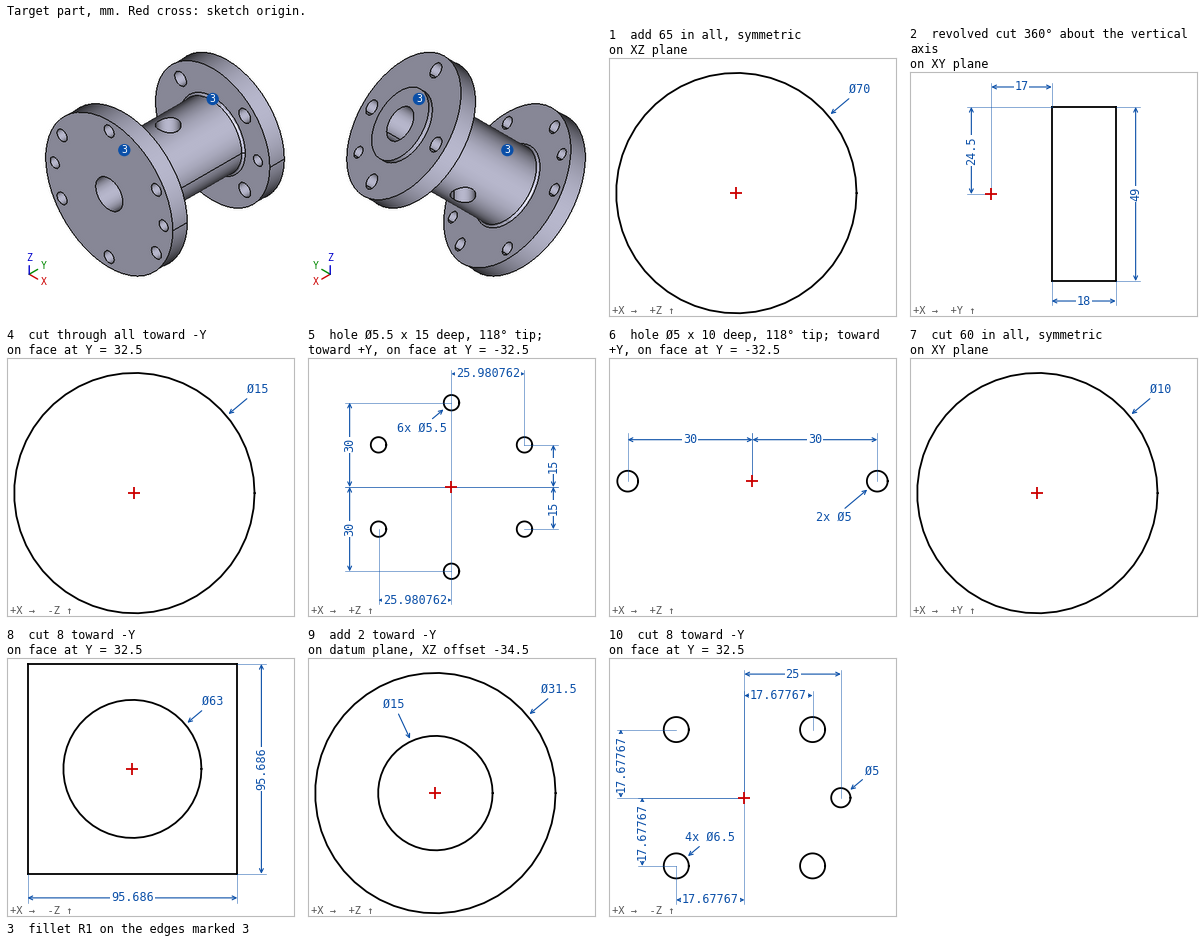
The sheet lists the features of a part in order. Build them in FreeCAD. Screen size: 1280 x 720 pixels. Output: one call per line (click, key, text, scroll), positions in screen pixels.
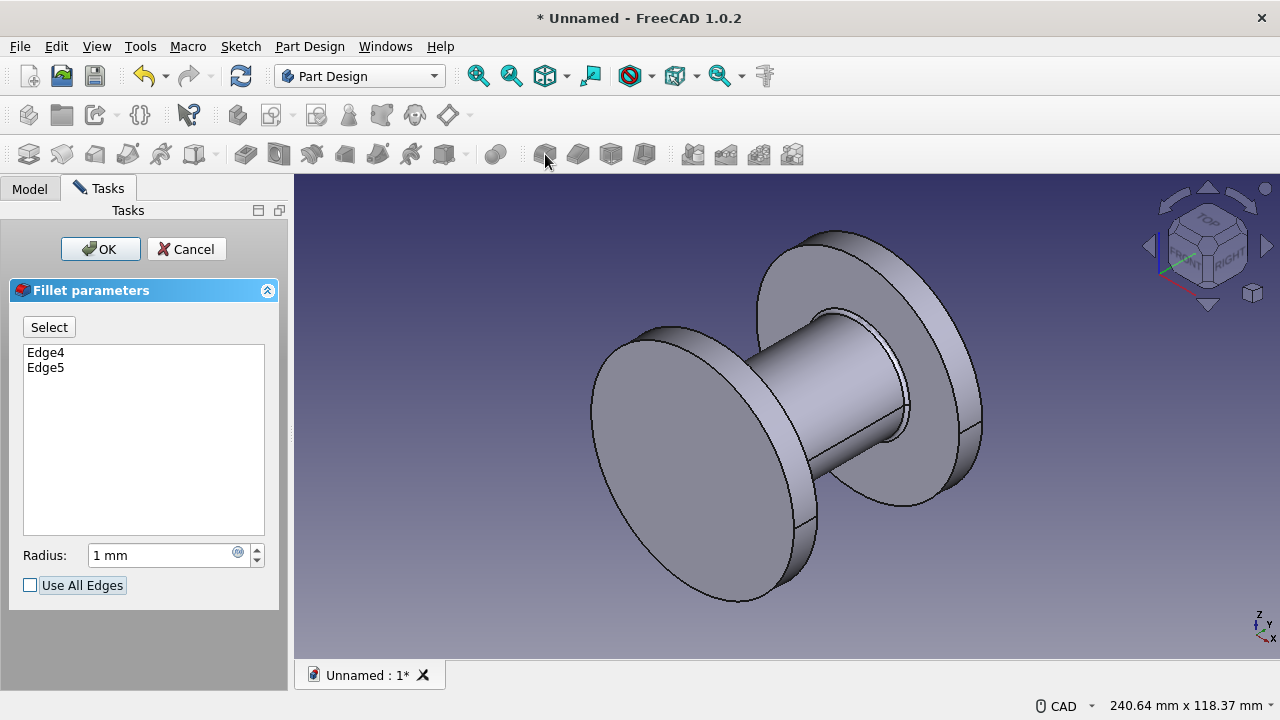
click(101, 249)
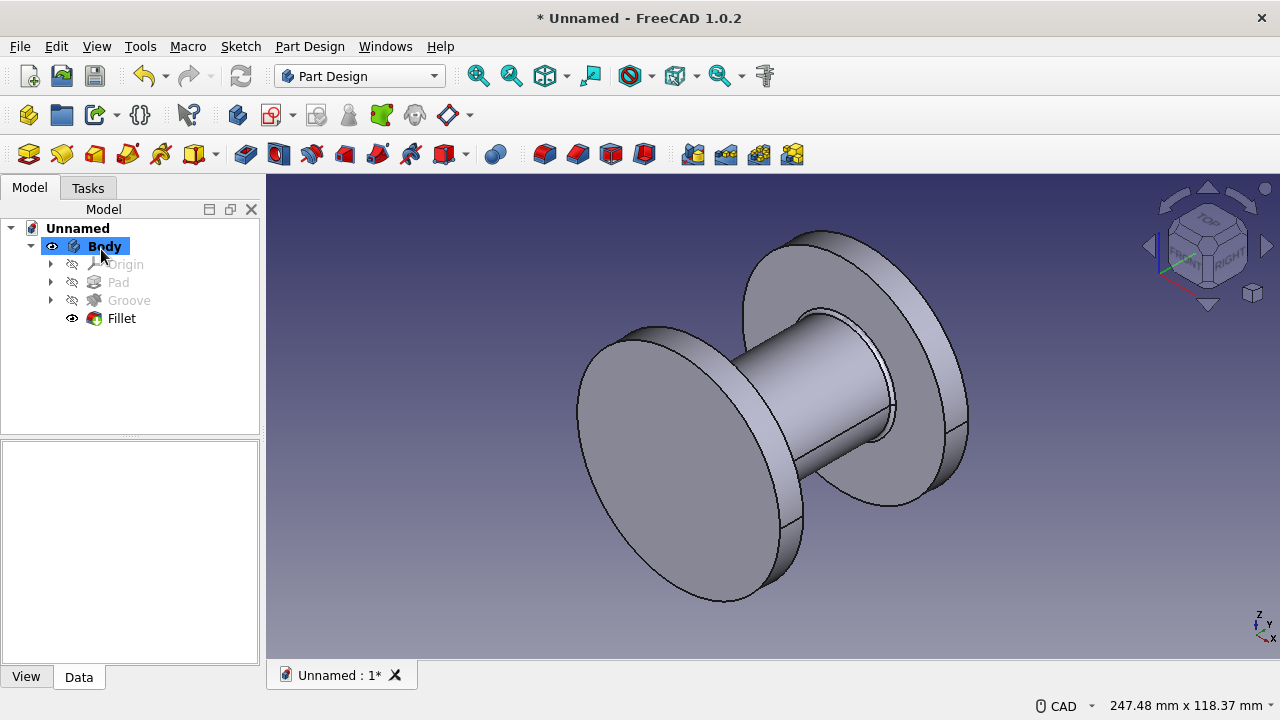
key(4)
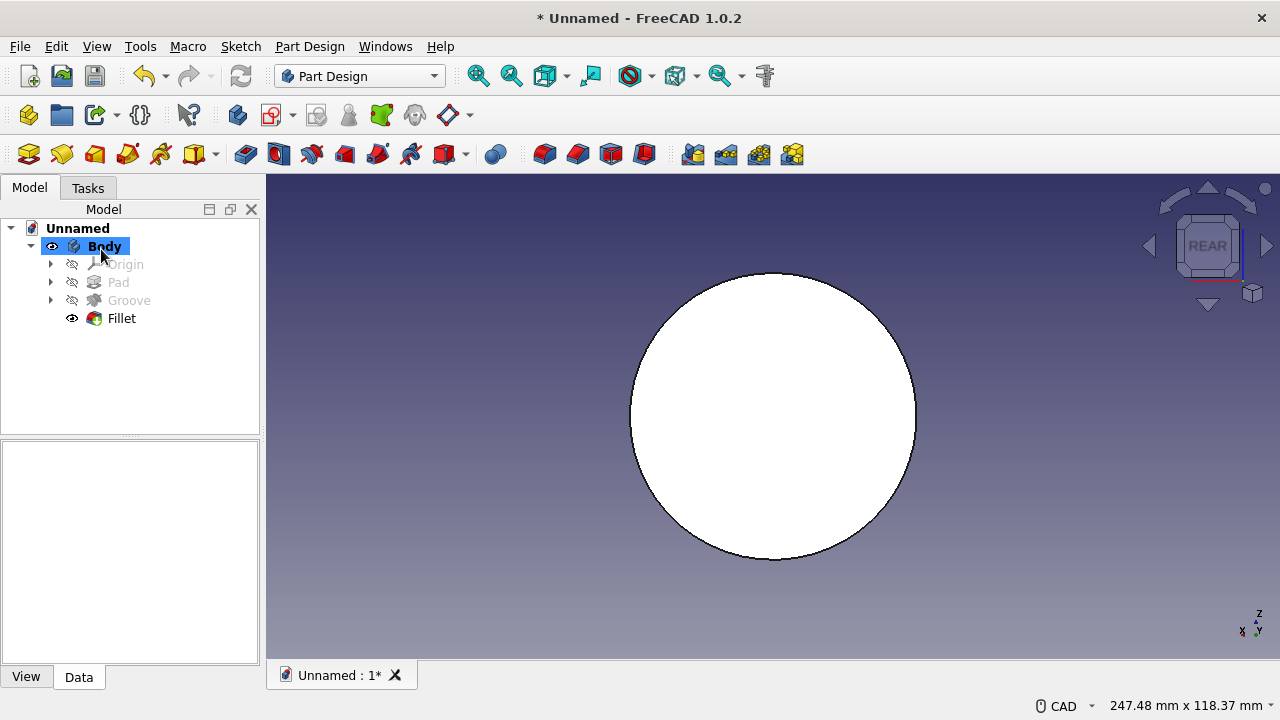
click(773, 415)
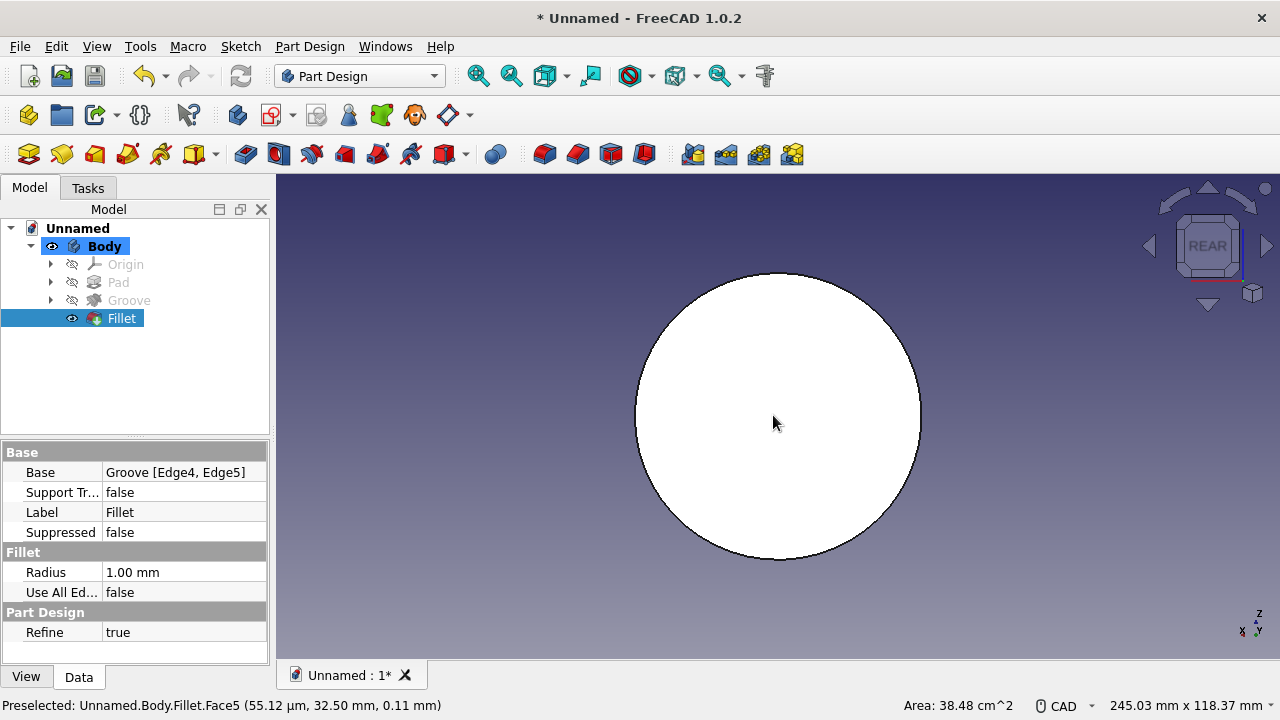
click(270, 116)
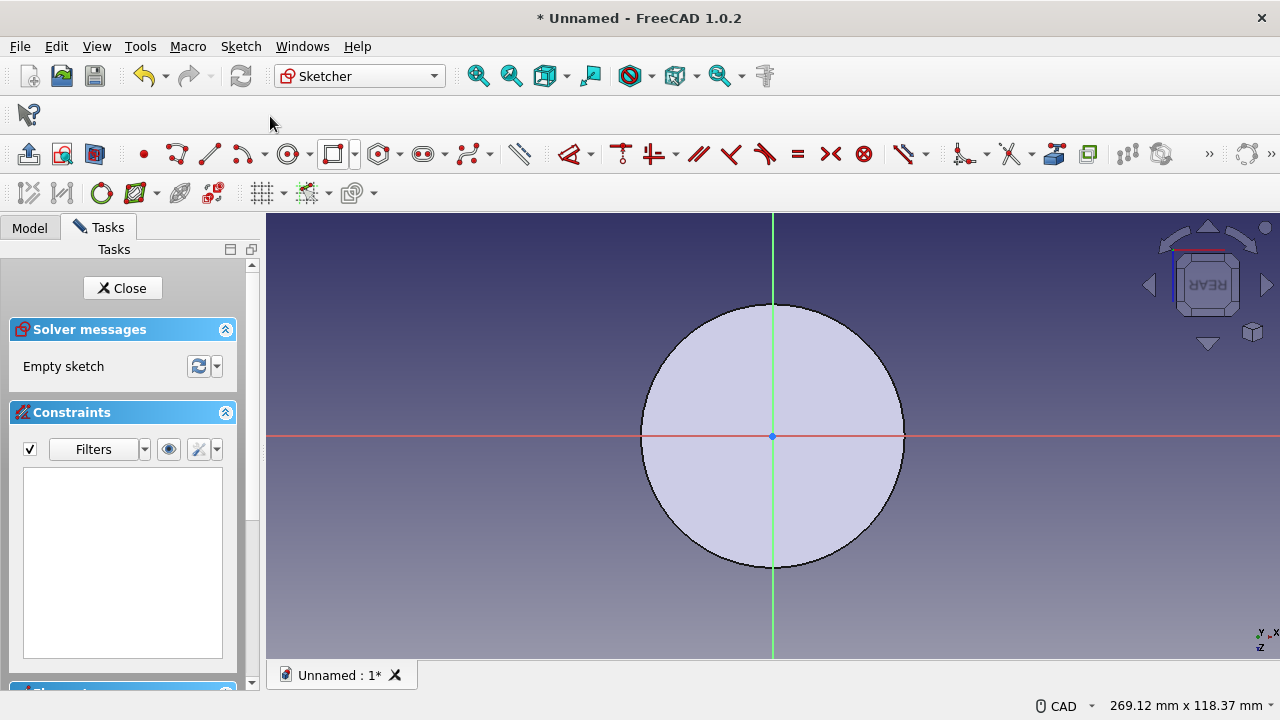
scroll(790, 436, up, 8)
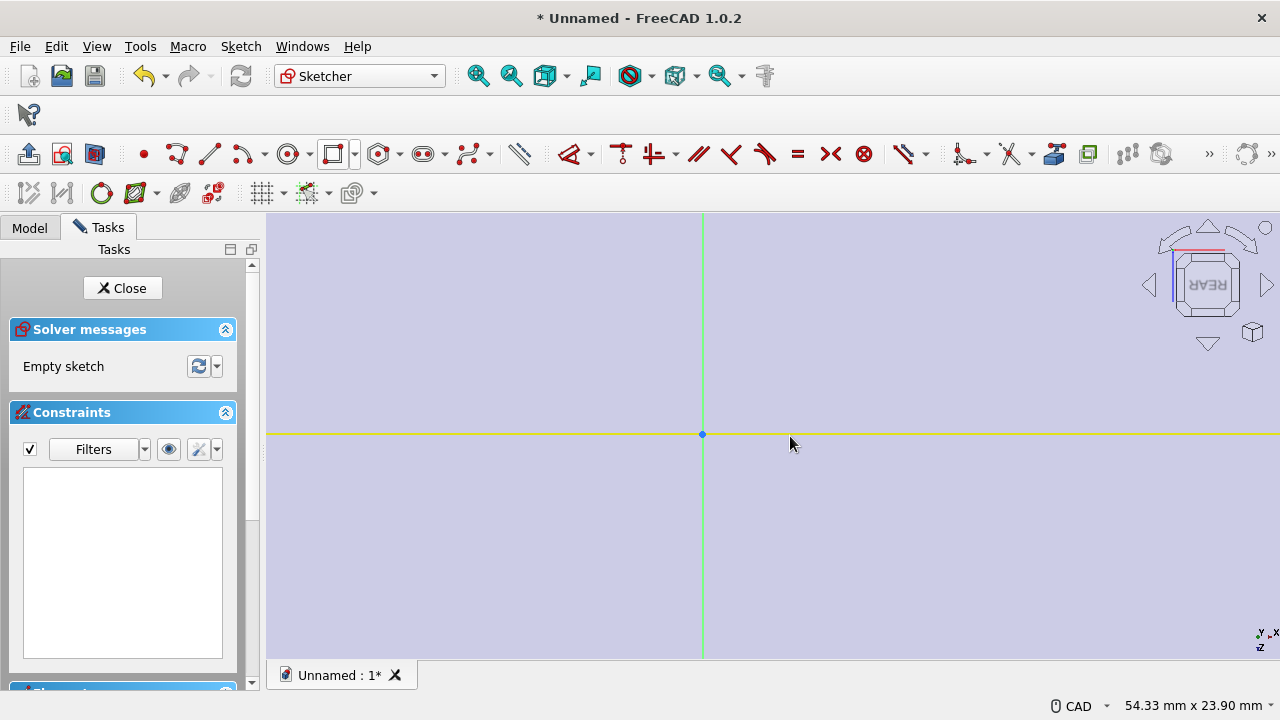
click(288, 154)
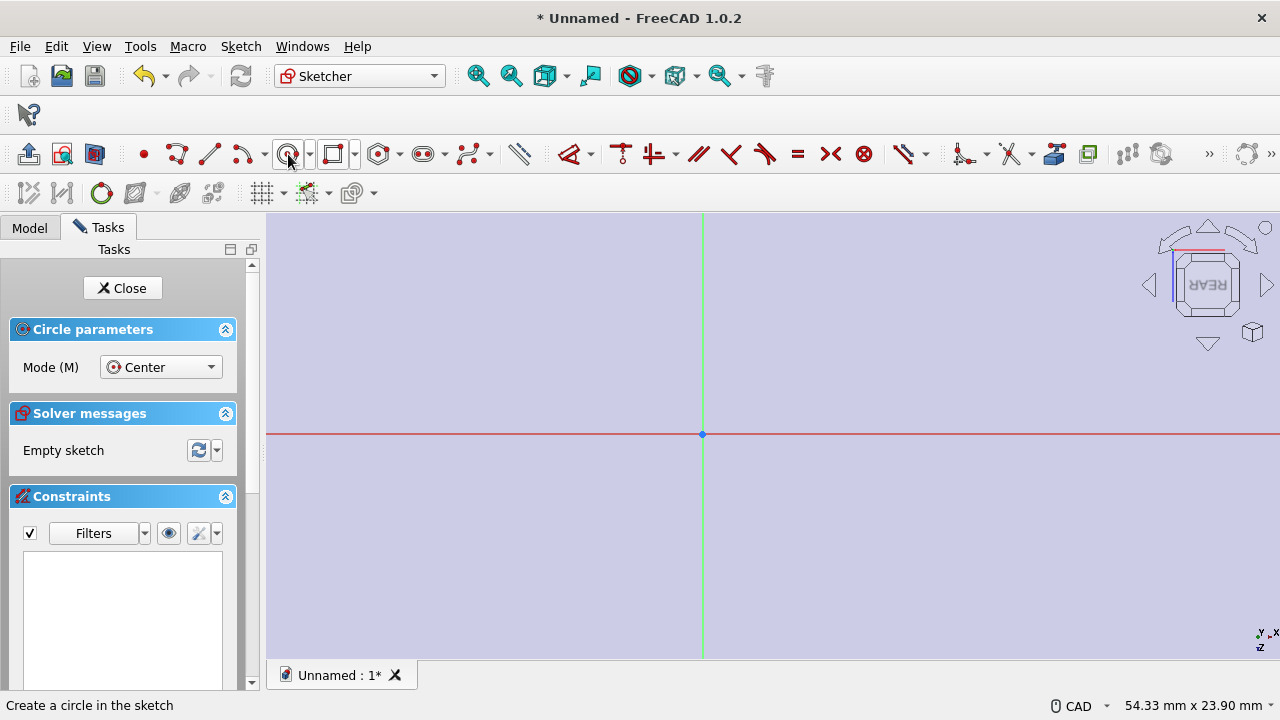
click(703, 434)
move(802, 335)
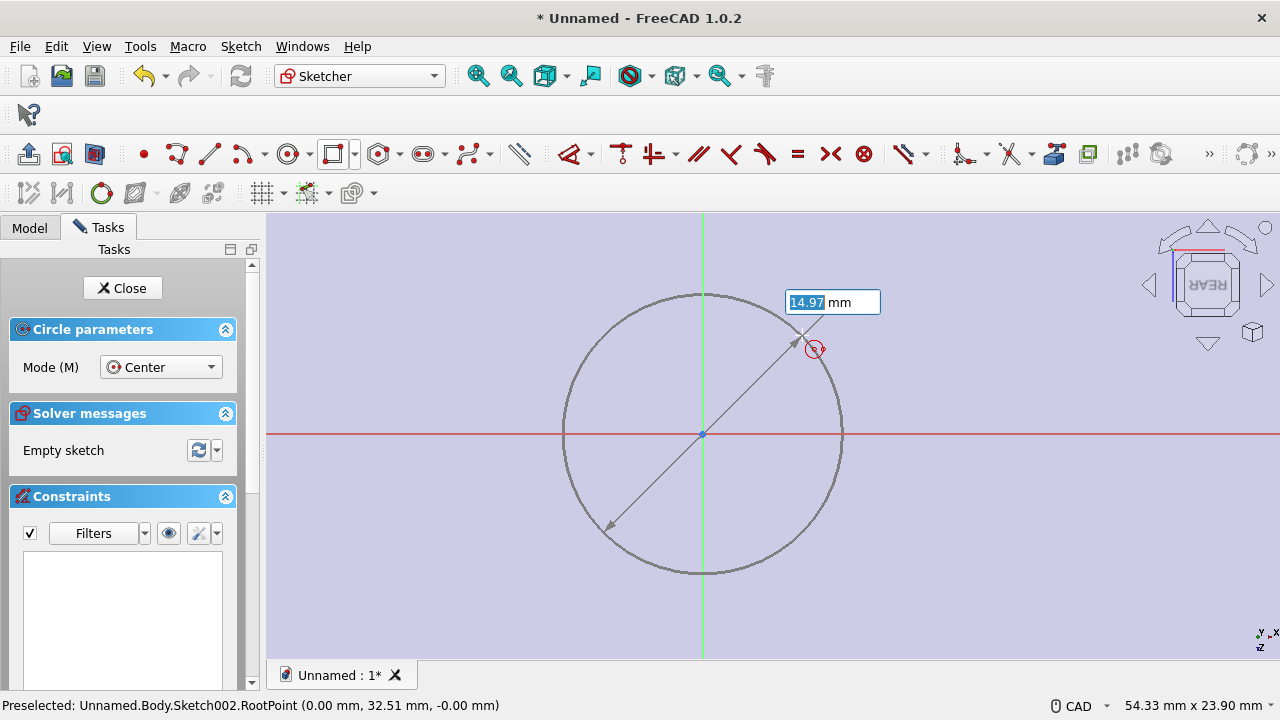
text(15)
key(Return)
key(Escape)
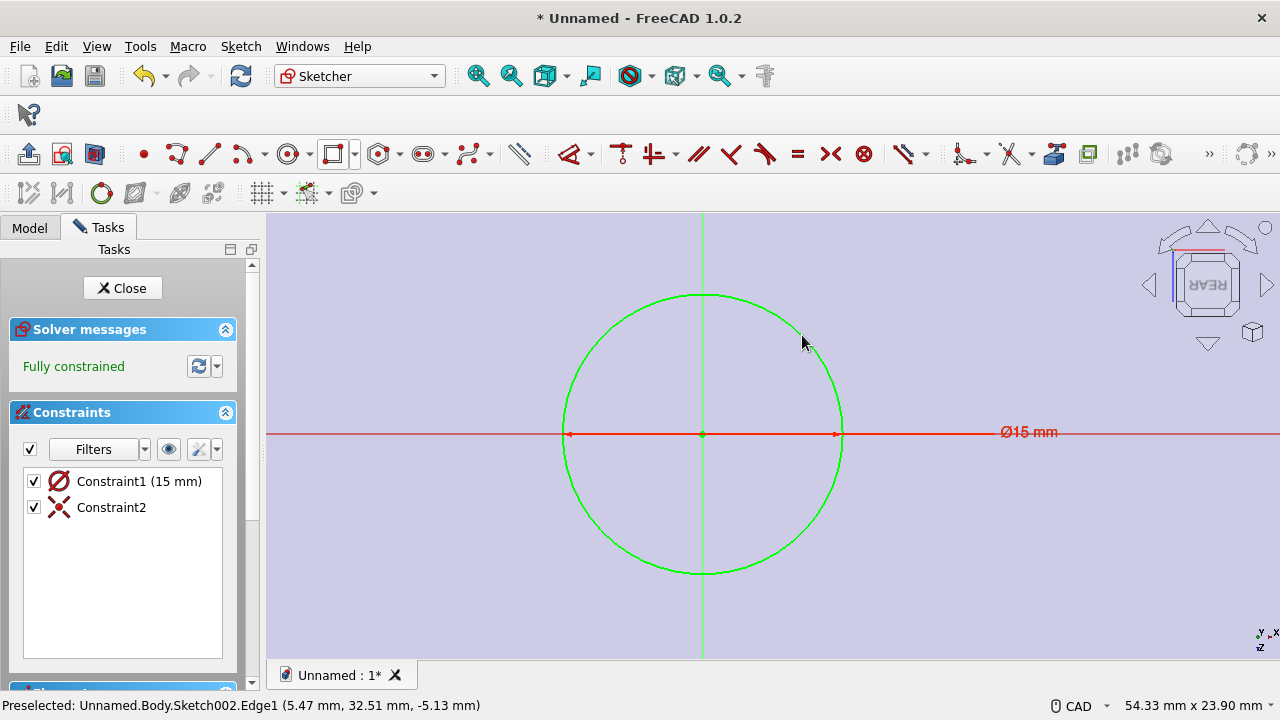
click(123, 288)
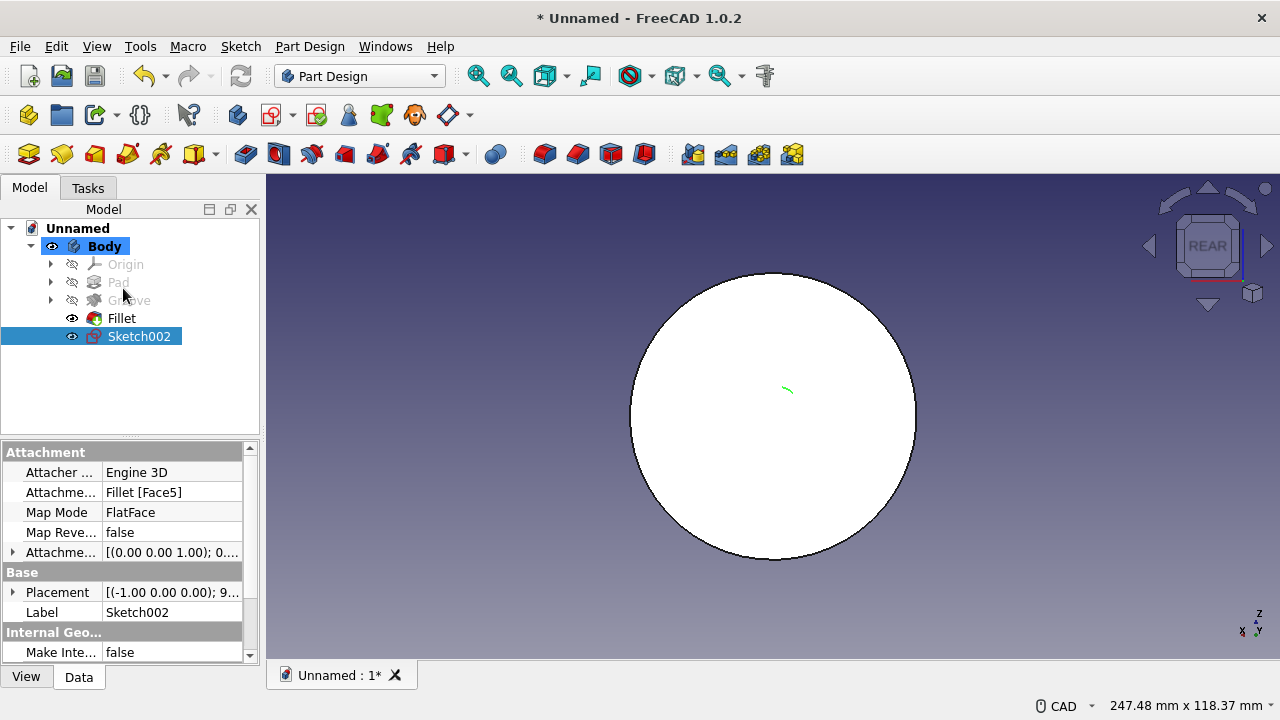
click(246, 154)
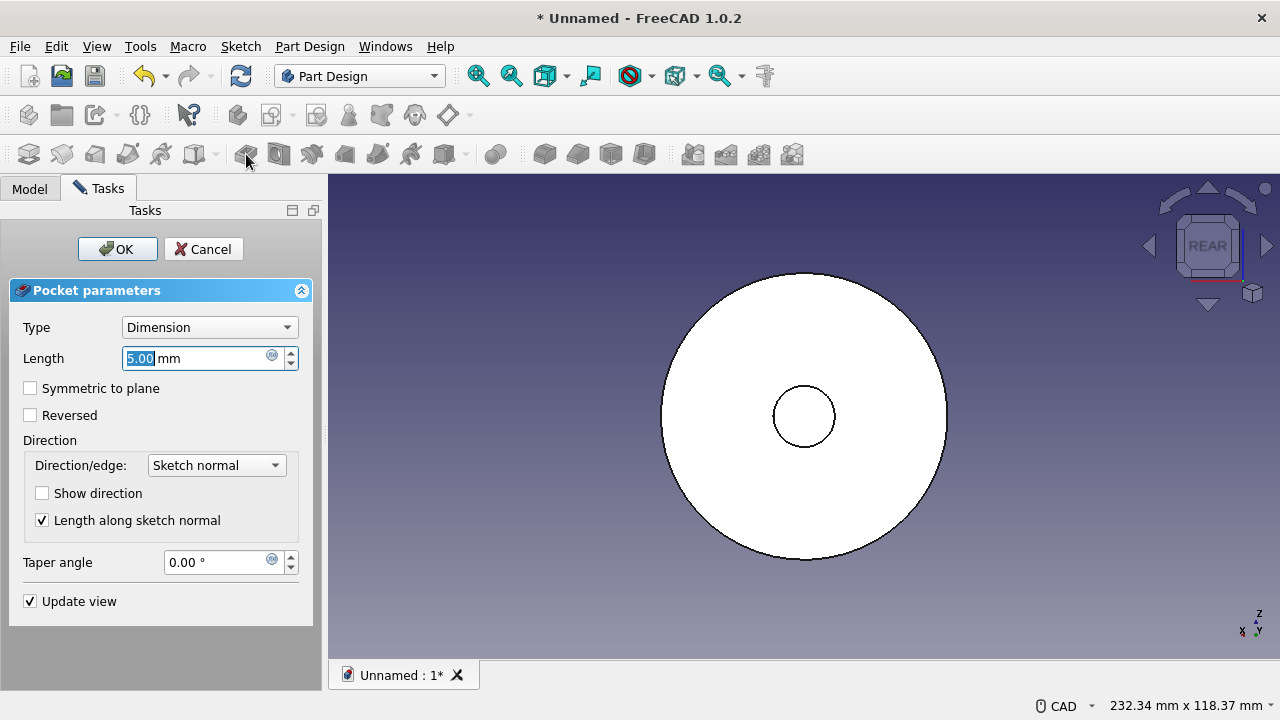
click(210, 328)